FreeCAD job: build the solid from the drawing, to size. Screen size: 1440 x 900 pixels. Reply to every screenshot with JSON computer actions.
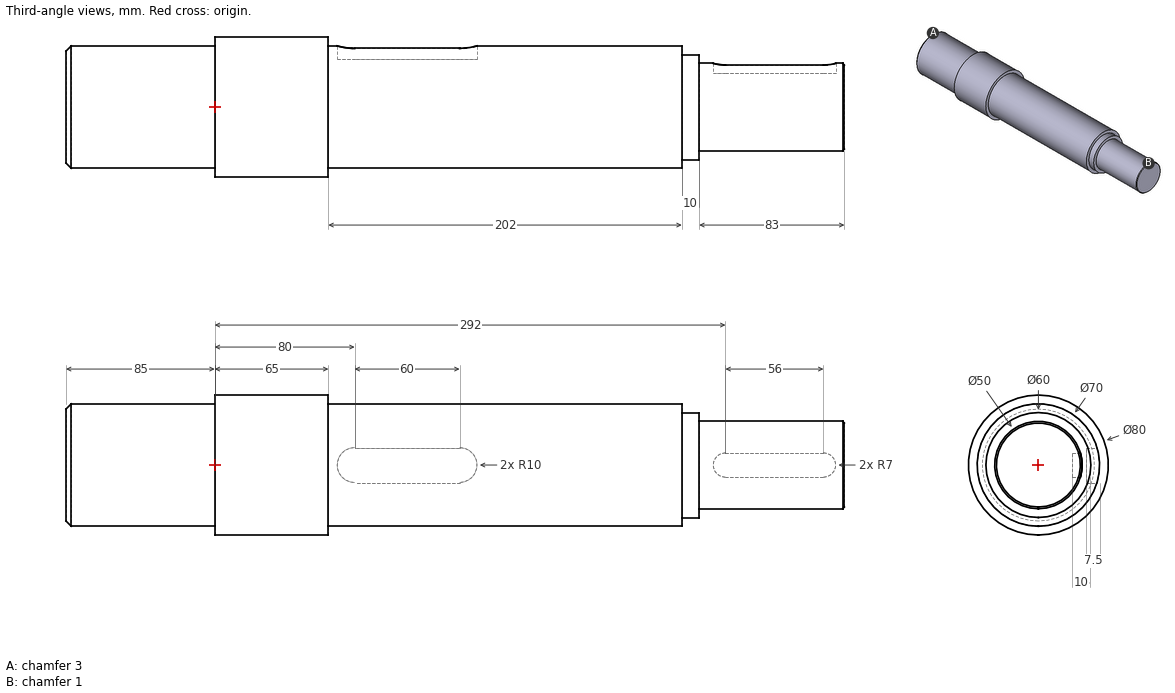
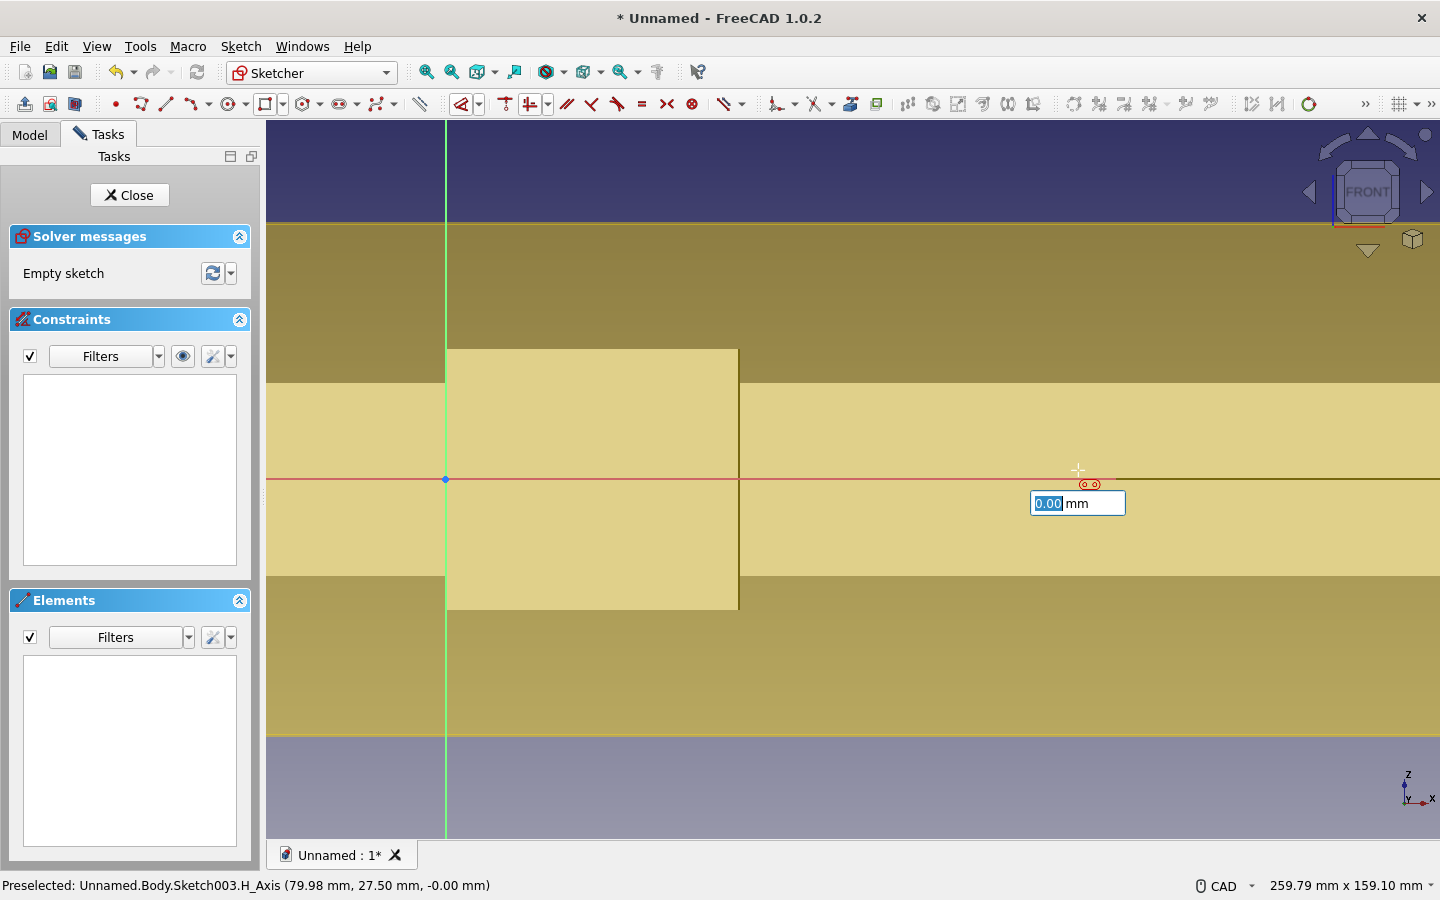
{"action": "left_click", "coordinate": [943, 434]}
{"action": "key", "text": "Escape"}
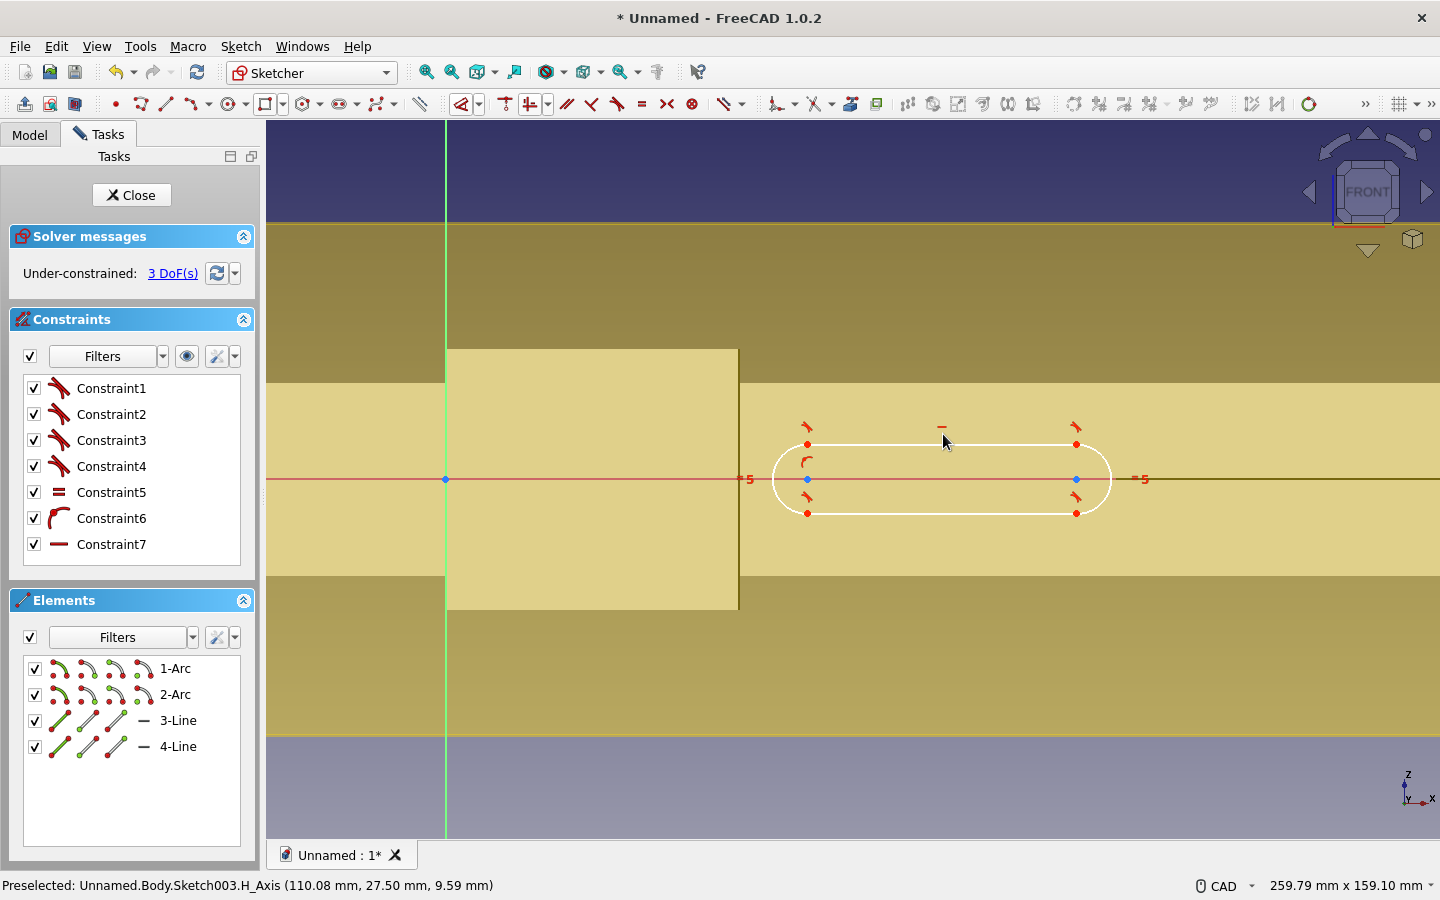
{"action": "key", "text": "d"}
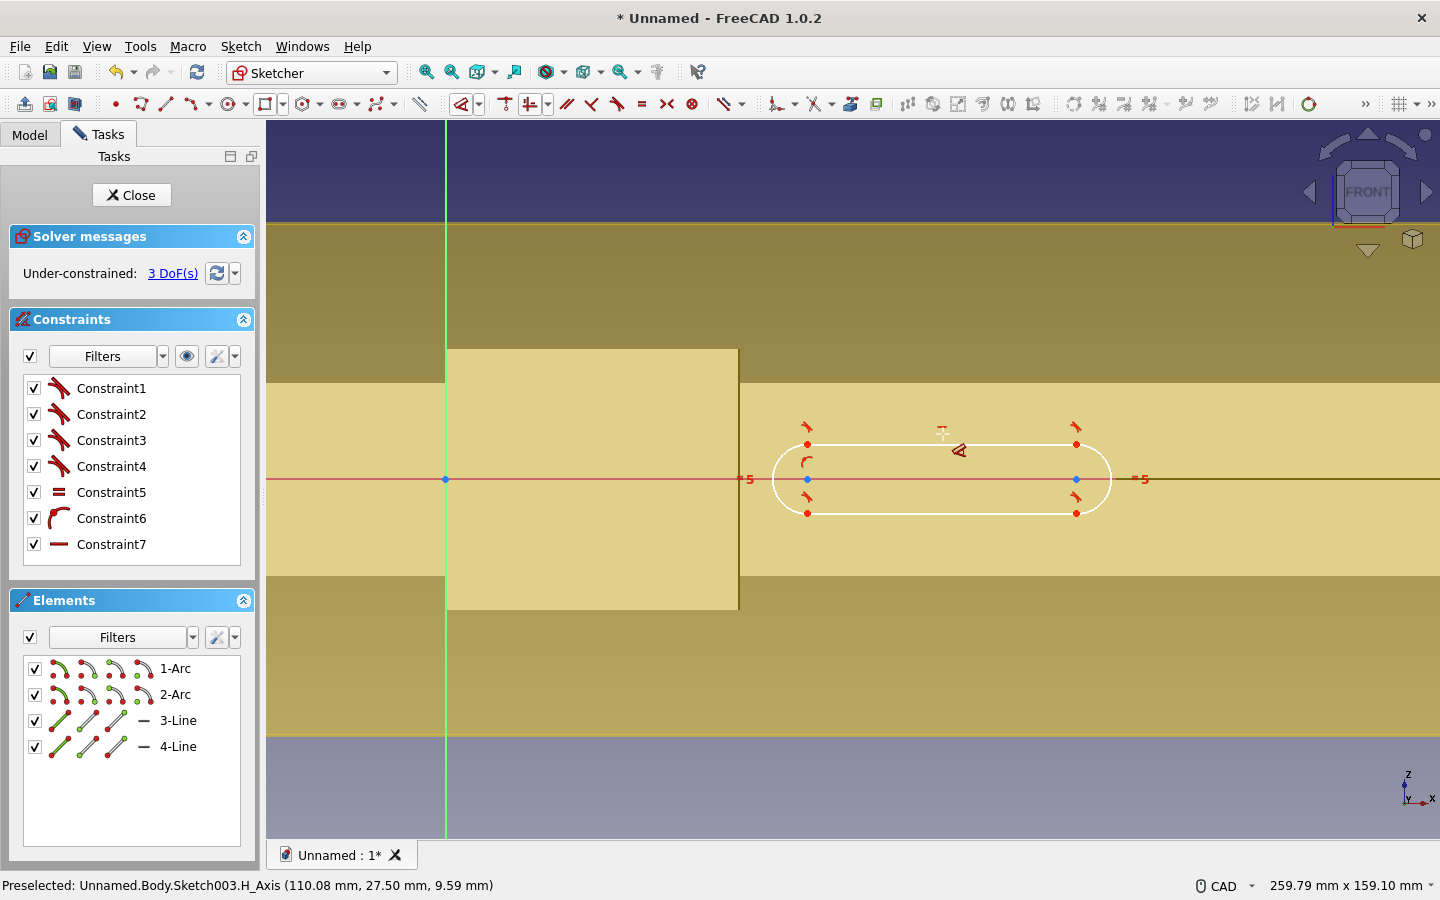
{"action": "left_click", "coordinate": [780, 459]}
{"action": "left_click", "coordinate": [754, 440]}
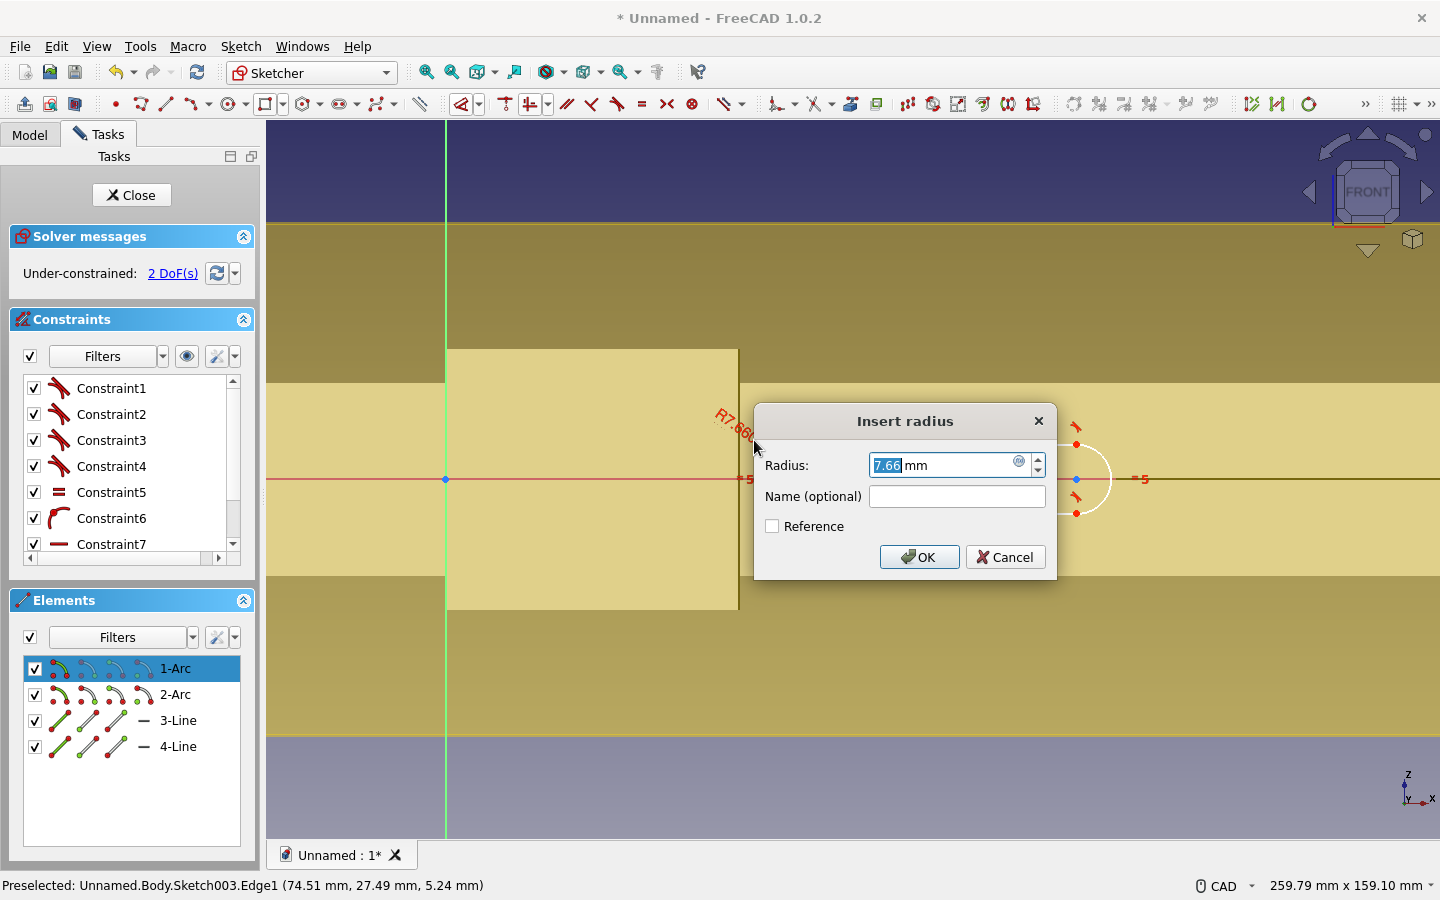
{"action": "type", "text": "10"}
{"action": "key", "text": "Return"}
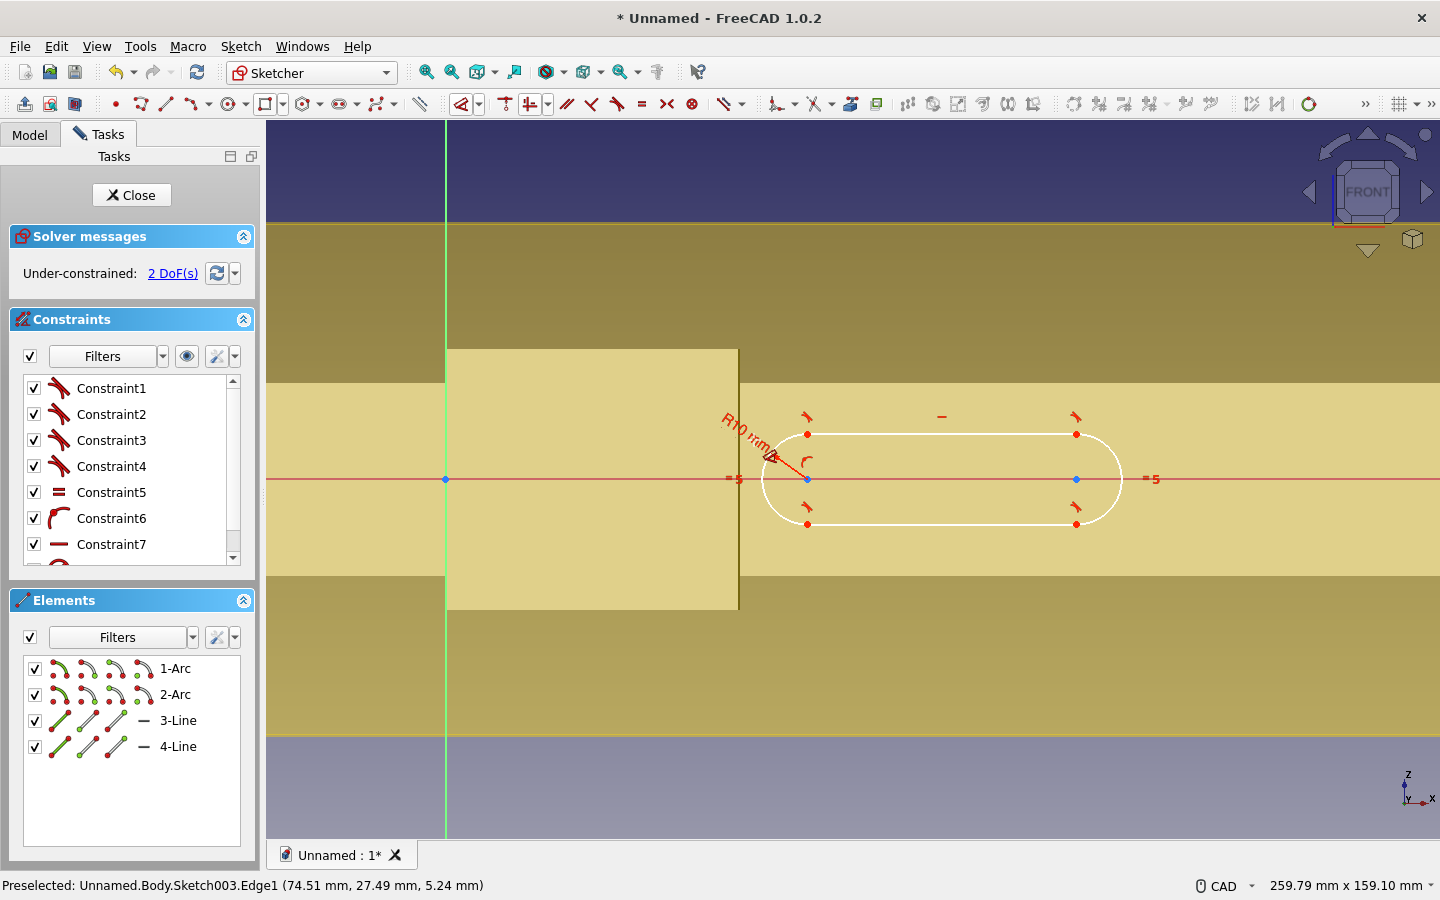
{"action": "left_click", "coordinate": [888, 434]}
{"action": "left_click", "coordinate": [942, 400]}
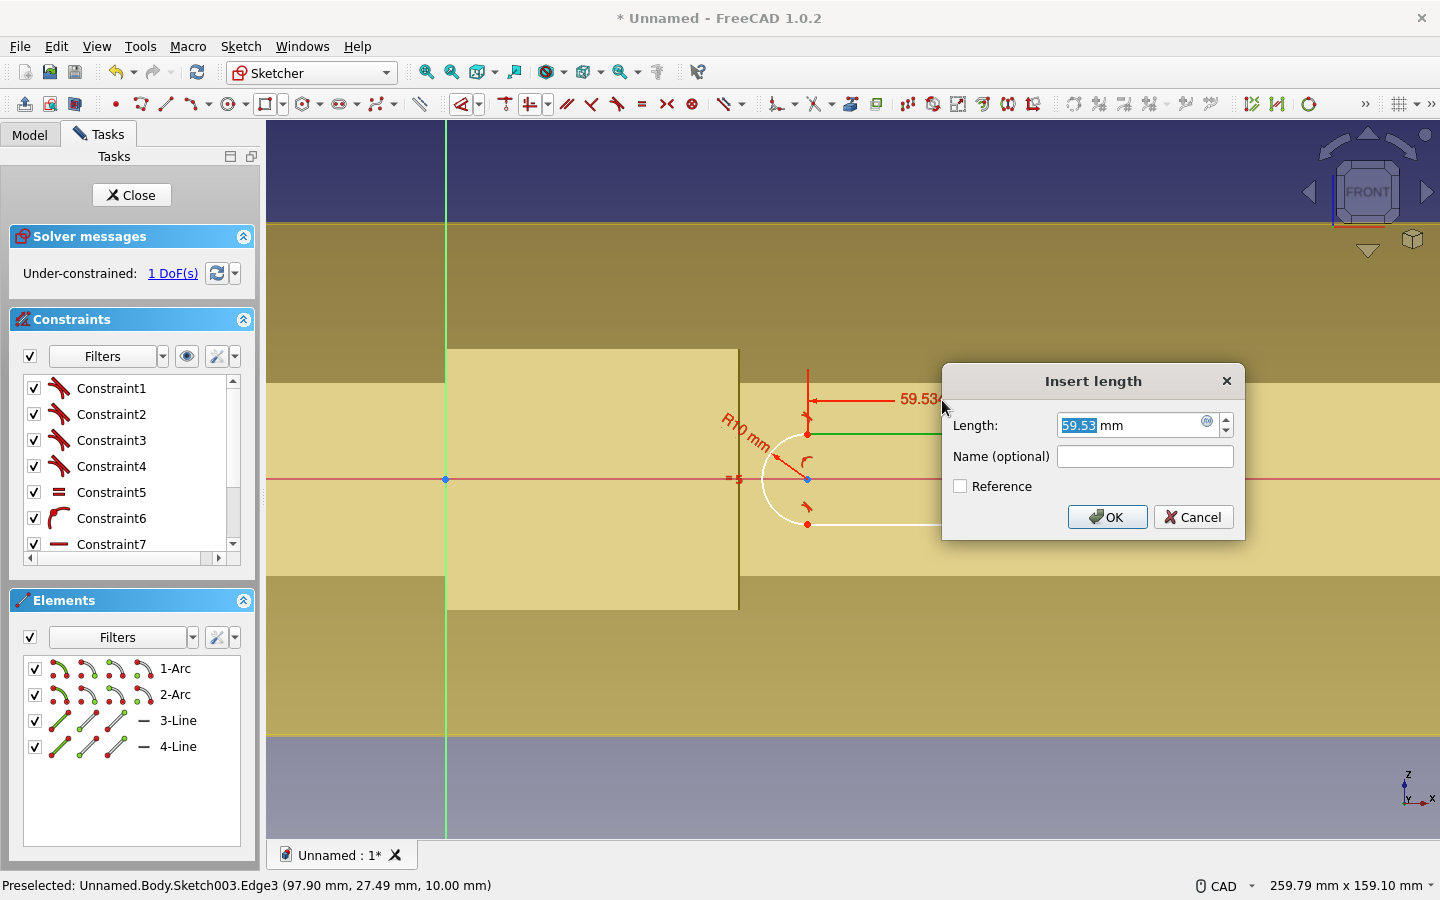
{"action": "type", "text": "60"}
{"action": "key", "text": "Return"}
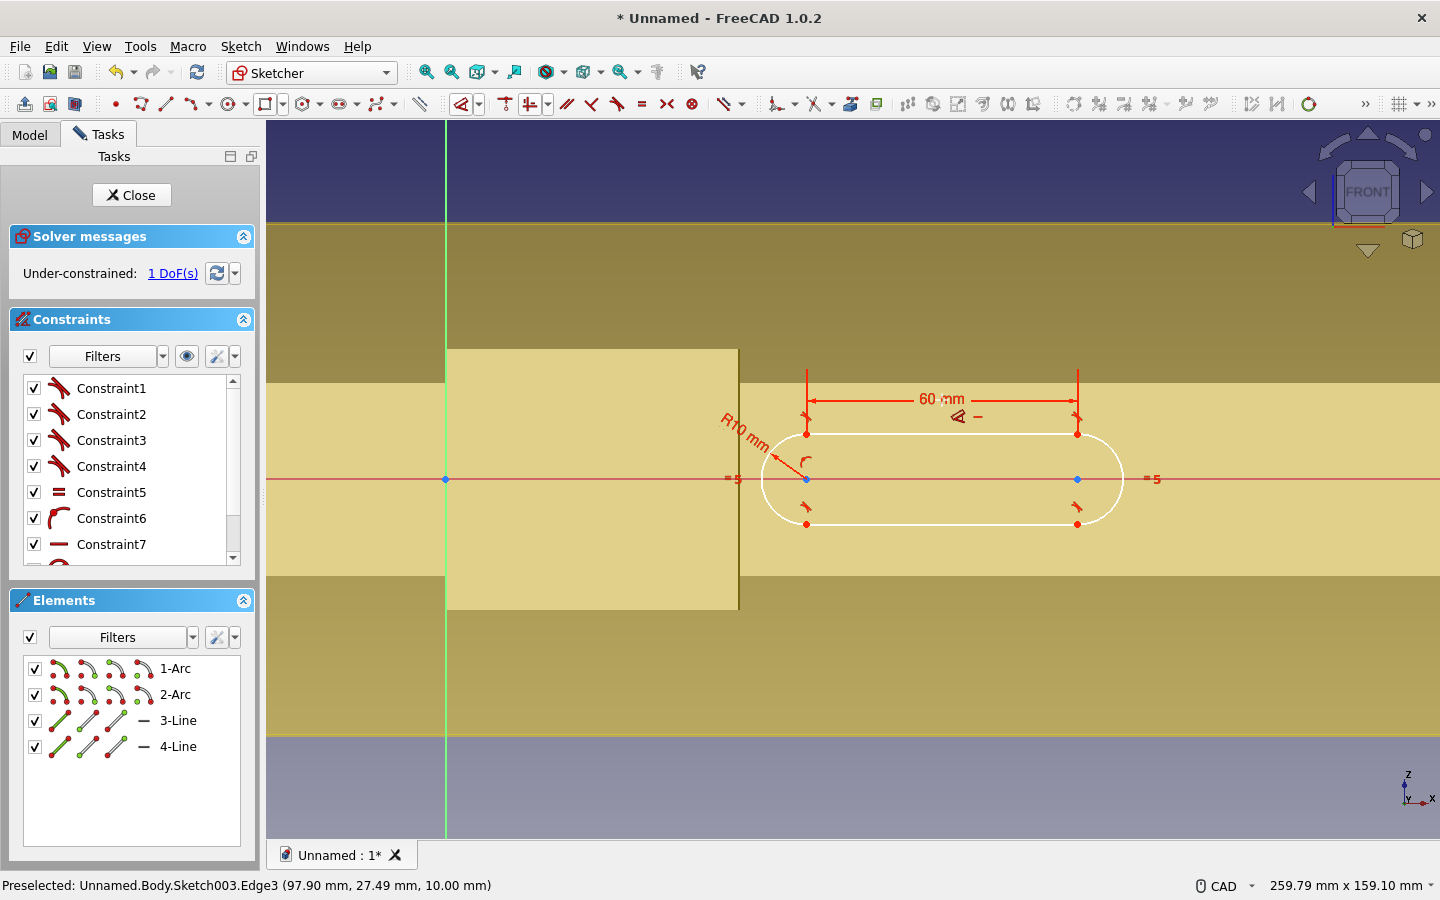
{"action": "left_click", "coordinate": [807, 434]}
{"action": "left_click", "coordinate": [626, 400]}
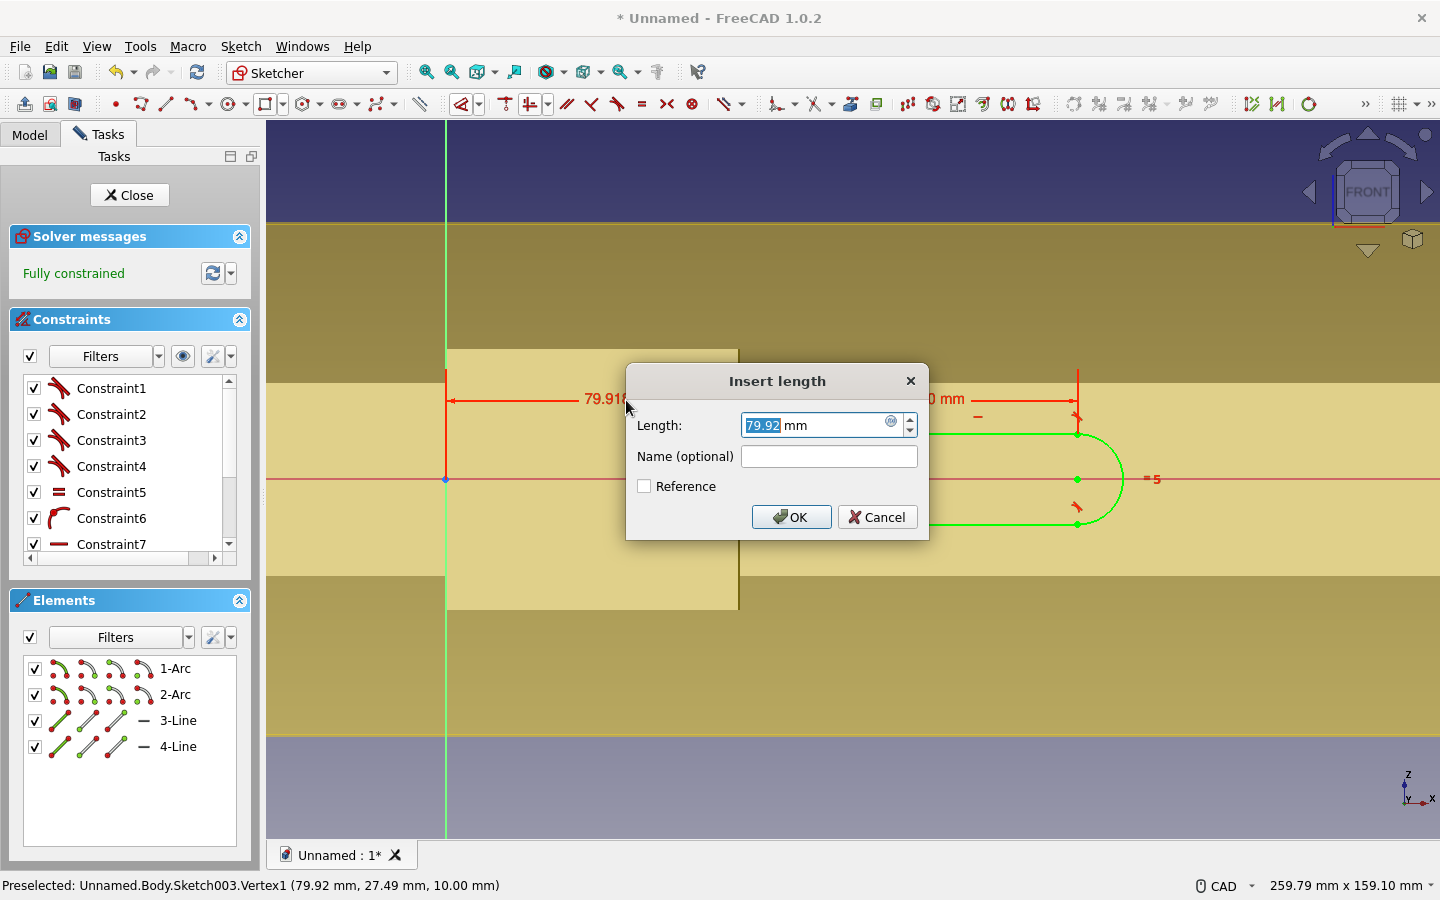
{"action": "type", "text": "80"}
{"action": "key", "text": "Return"}
{"action": "key", "text": "Escape"}